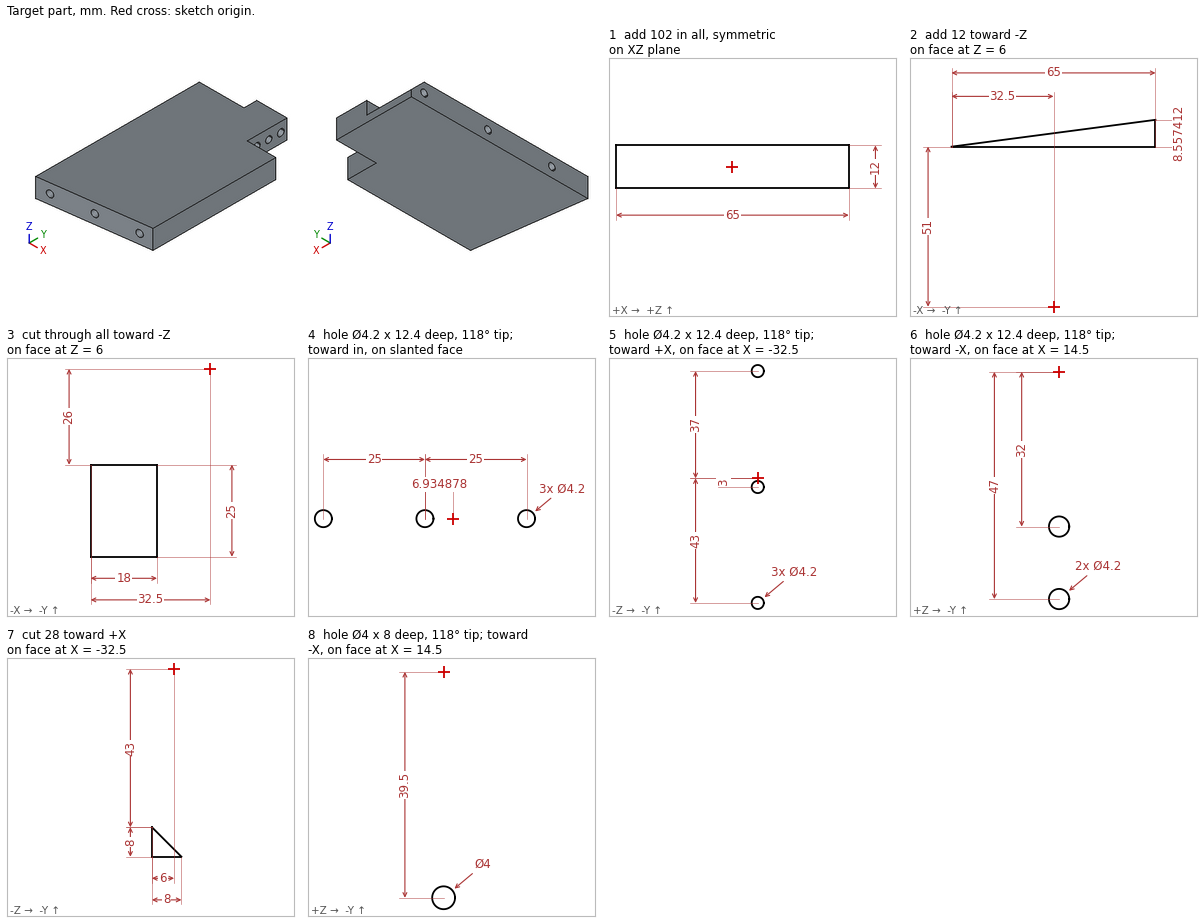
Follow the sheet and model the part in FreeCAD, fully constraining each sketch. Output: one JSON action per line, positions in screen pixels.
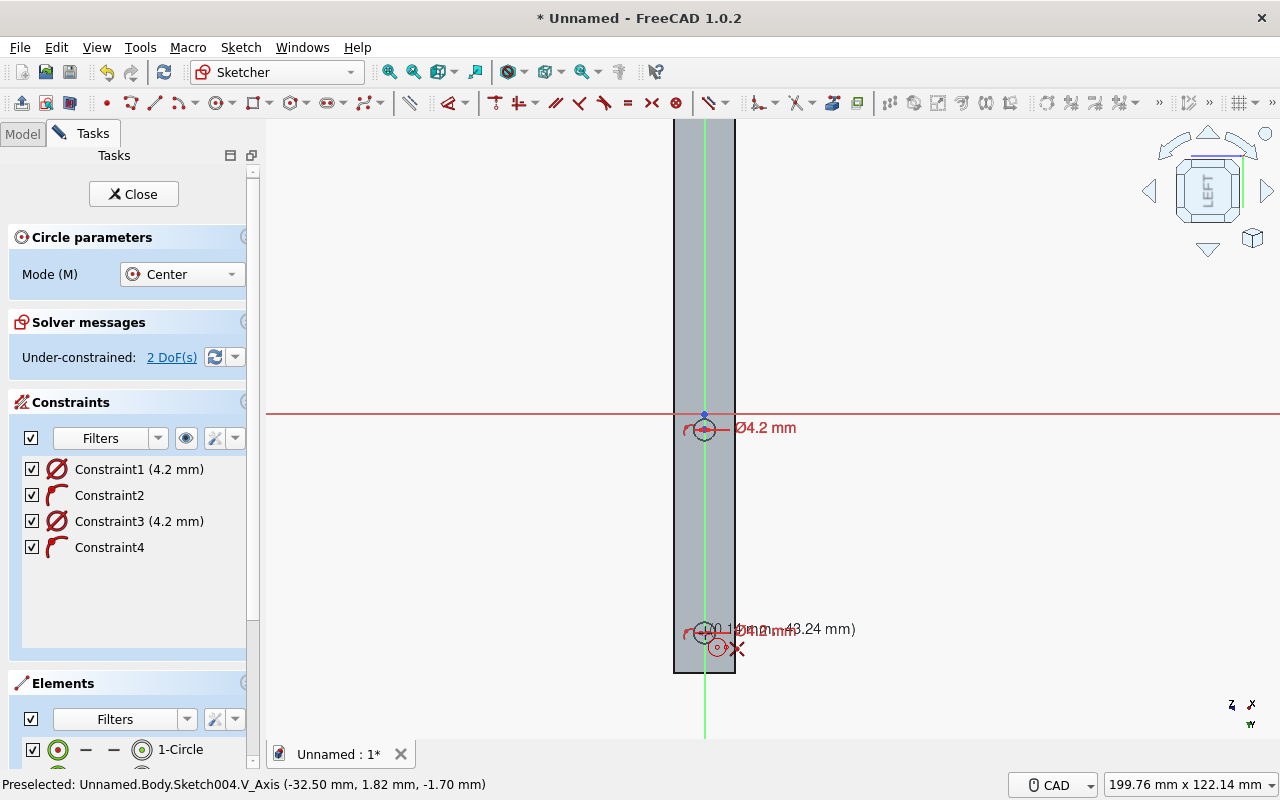
{"action": "scroll", "coordinate": [705, 227], "scroll_direction": "up", "scroll_amount": 4}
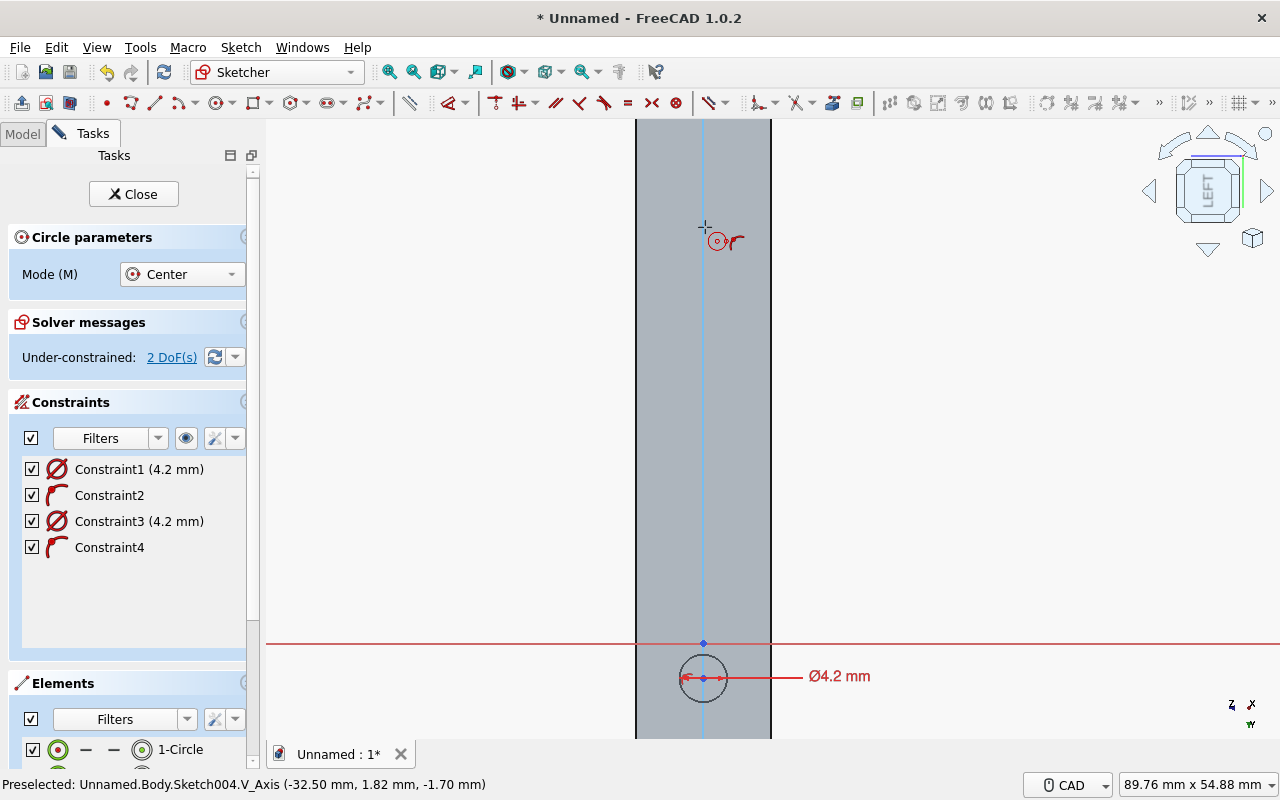
{"action": "left_click", "coordinate": [703, 226]}
{"action": "mouse_move", "coordinate": [720, 209]}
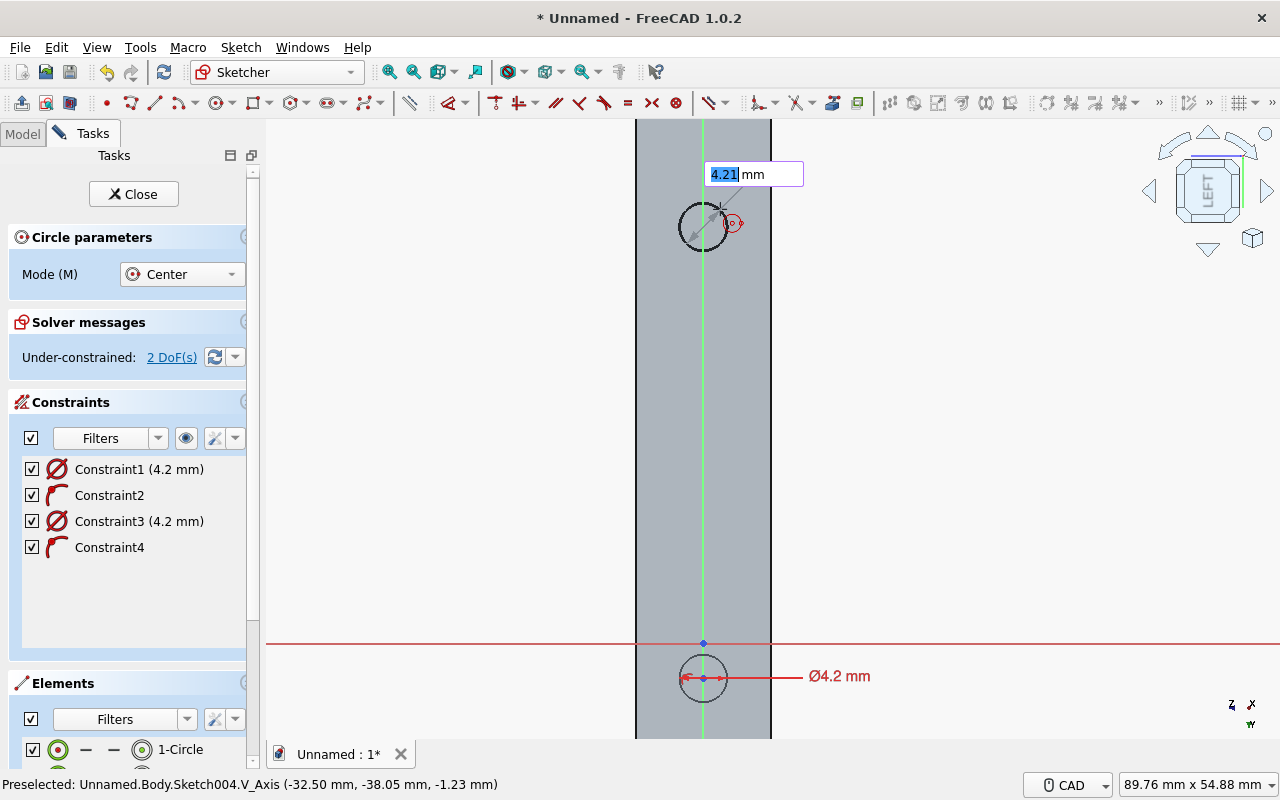
{"action": "type", "text": "4.2"}
{"action": "key", "text": "Return"}
{"action": "key", "text": "Escape"}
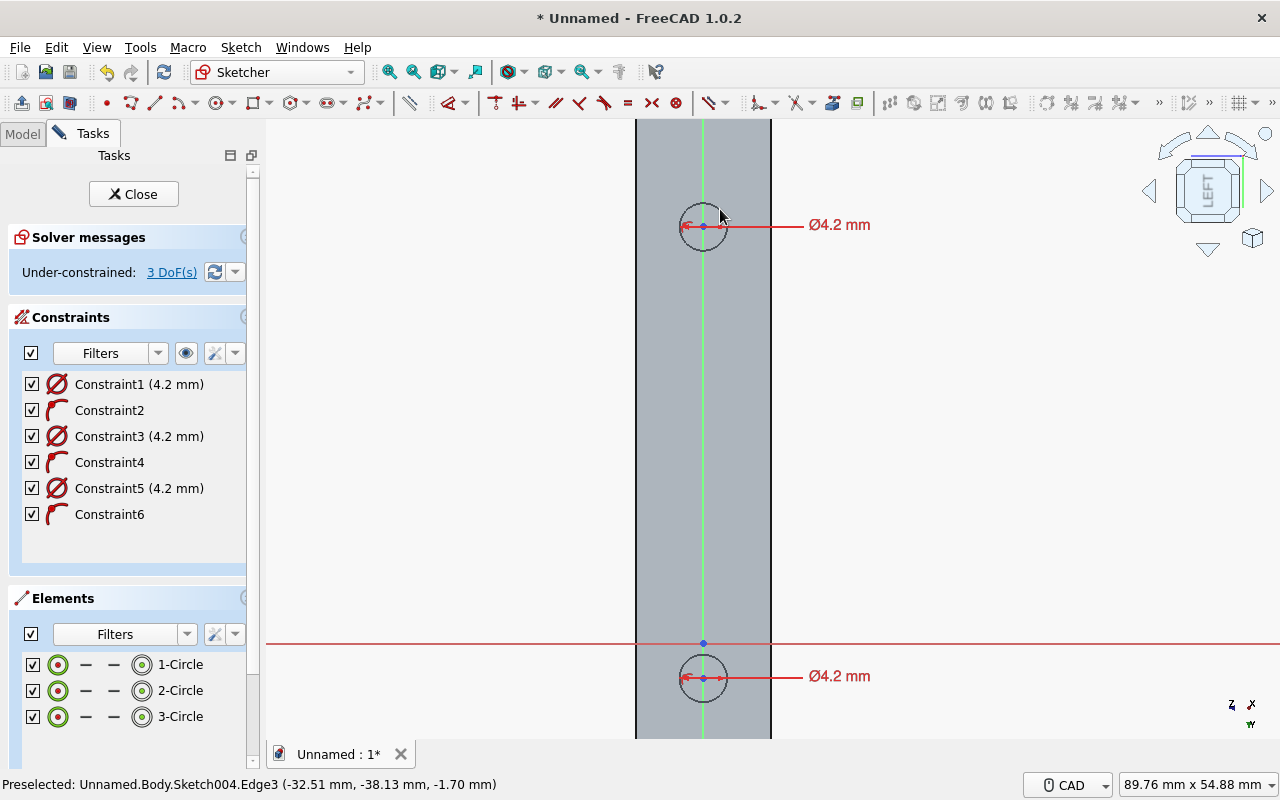
{"action": "key", "text": "d"}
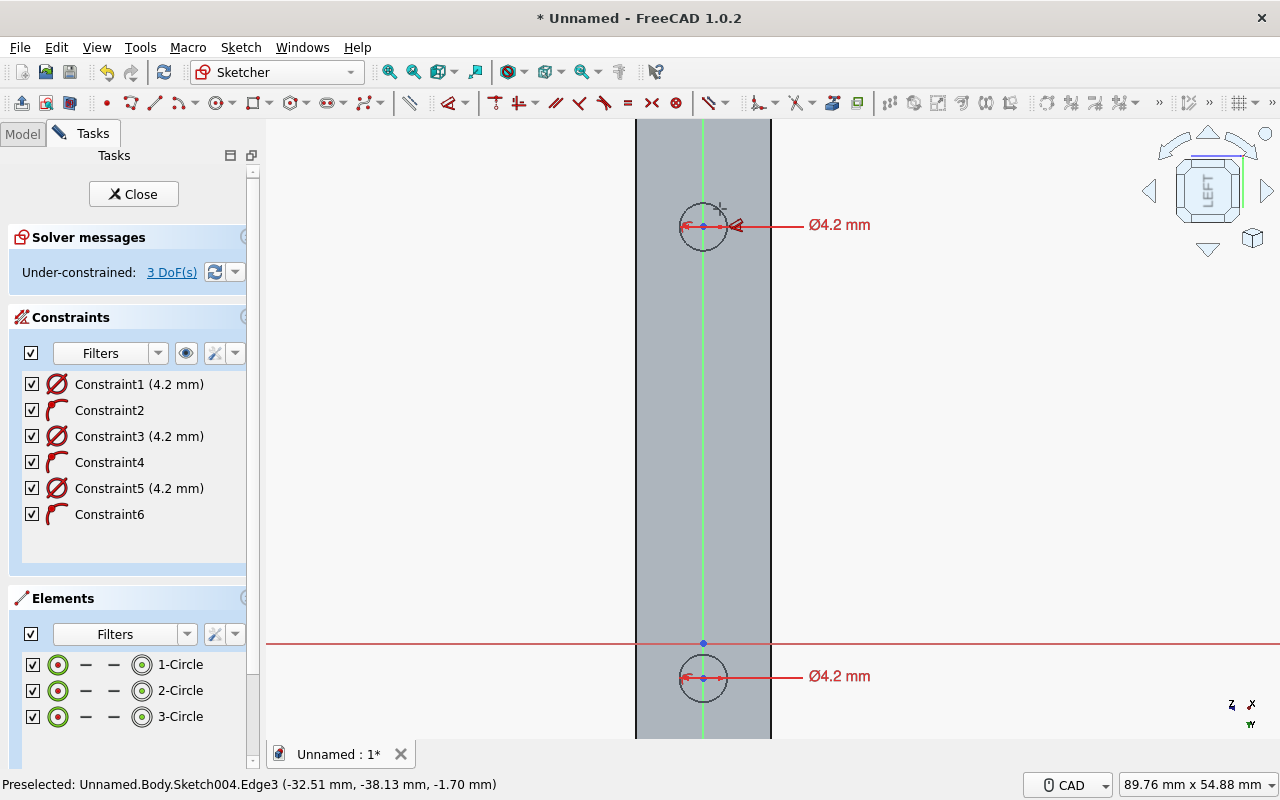
{"action": "left_click", "coordinate": [703, 678]}
{"action": "left_click", "coordinate": [737, 661]}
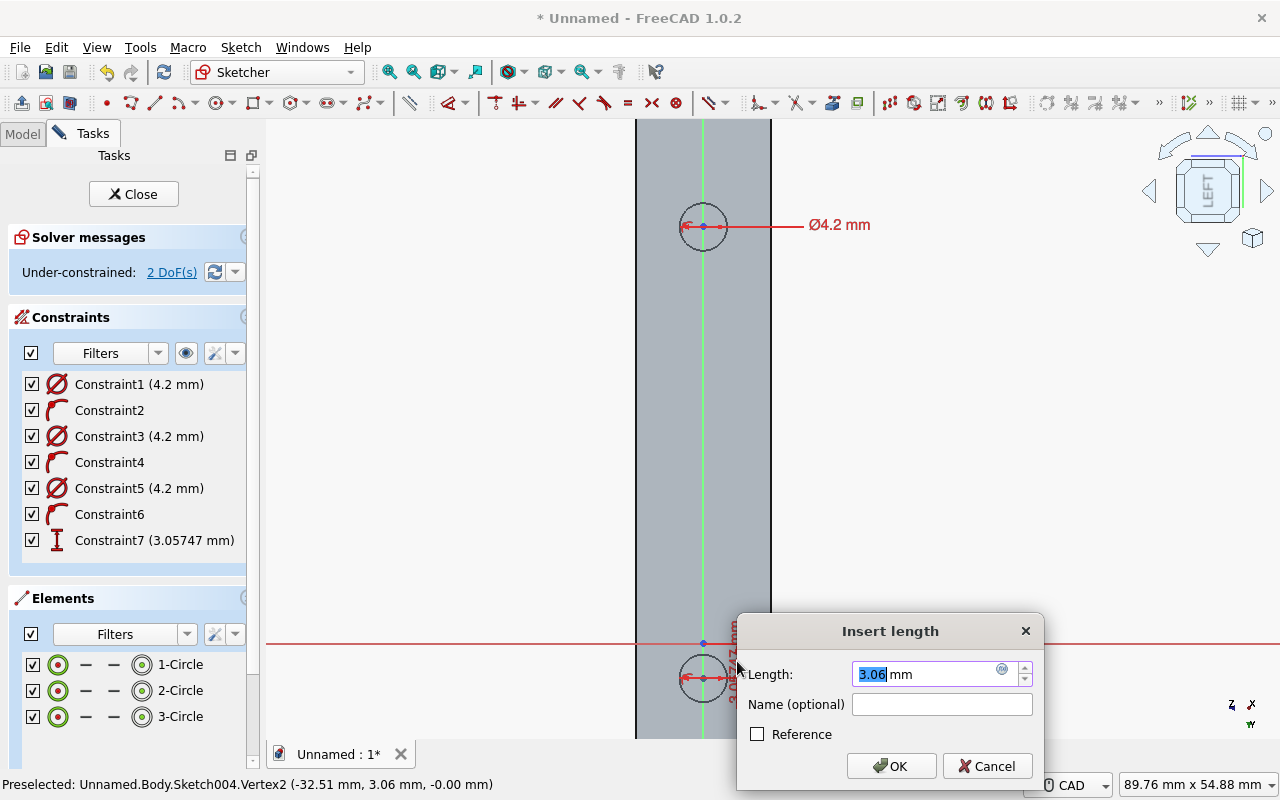
{"action": "type", "text": "3"}
{"action": "key", "text": "Return"}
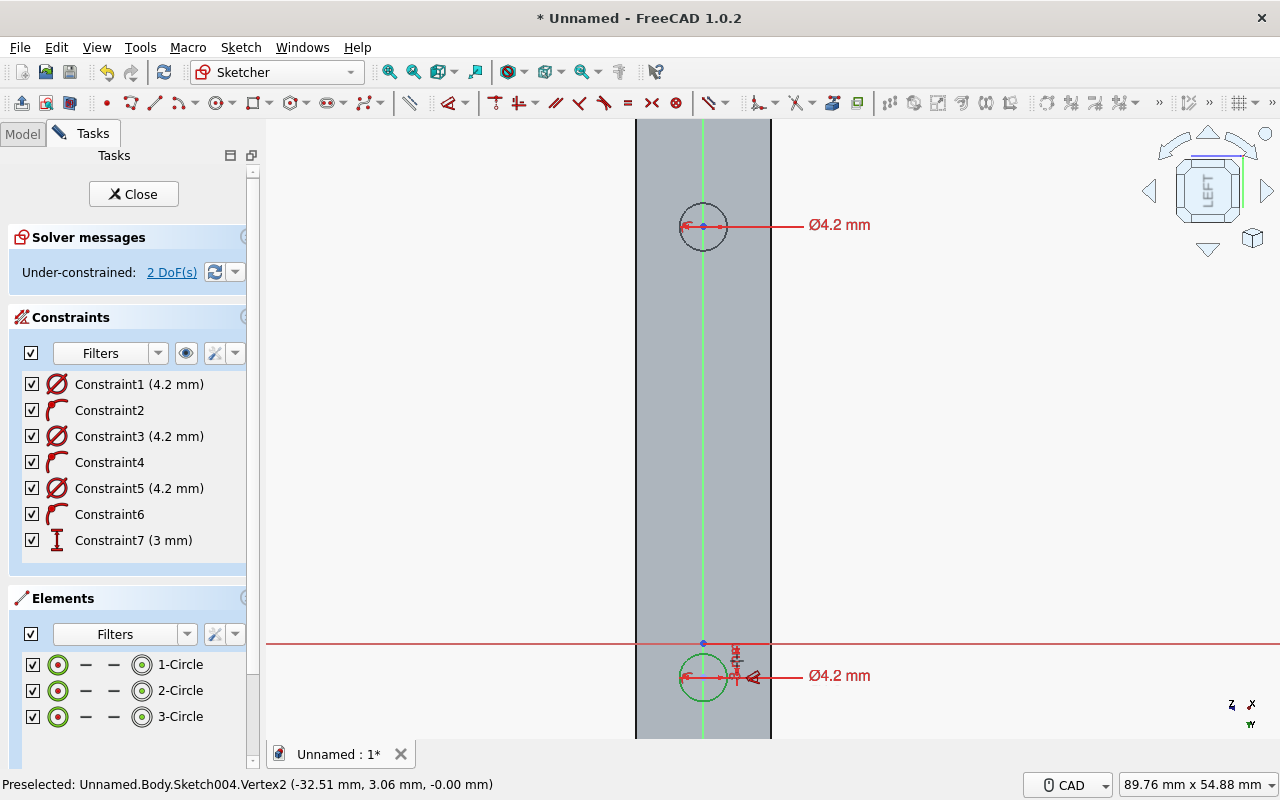
{"action": "scroll", "coordinate": [705, 226], "scroll_direction": "down", "scroll_amount": 4}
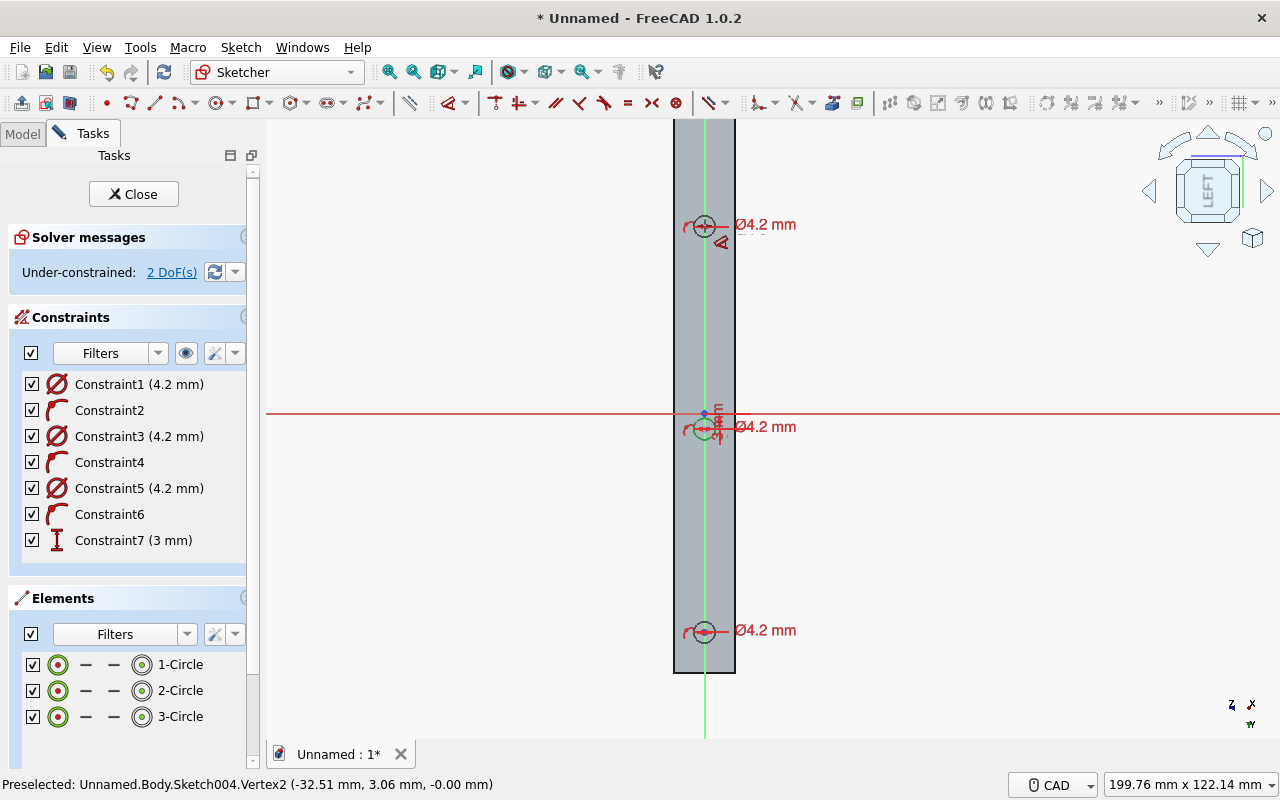
{"action": "left_click", "coordinate": [705, 632]}
{"action": "left_click", "coordinate": [739, 523]}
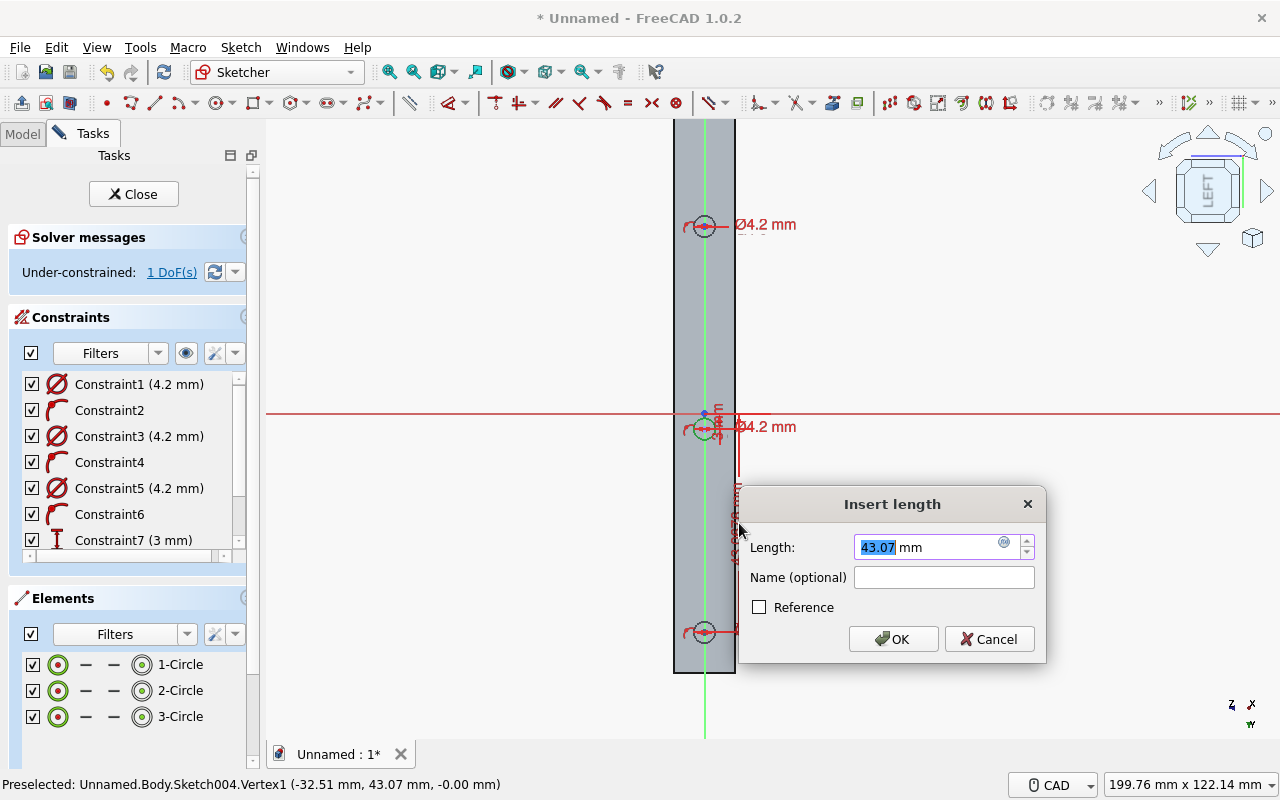
{"action": "type", "text": "43"}
{"action": "key", "text": "Return"}